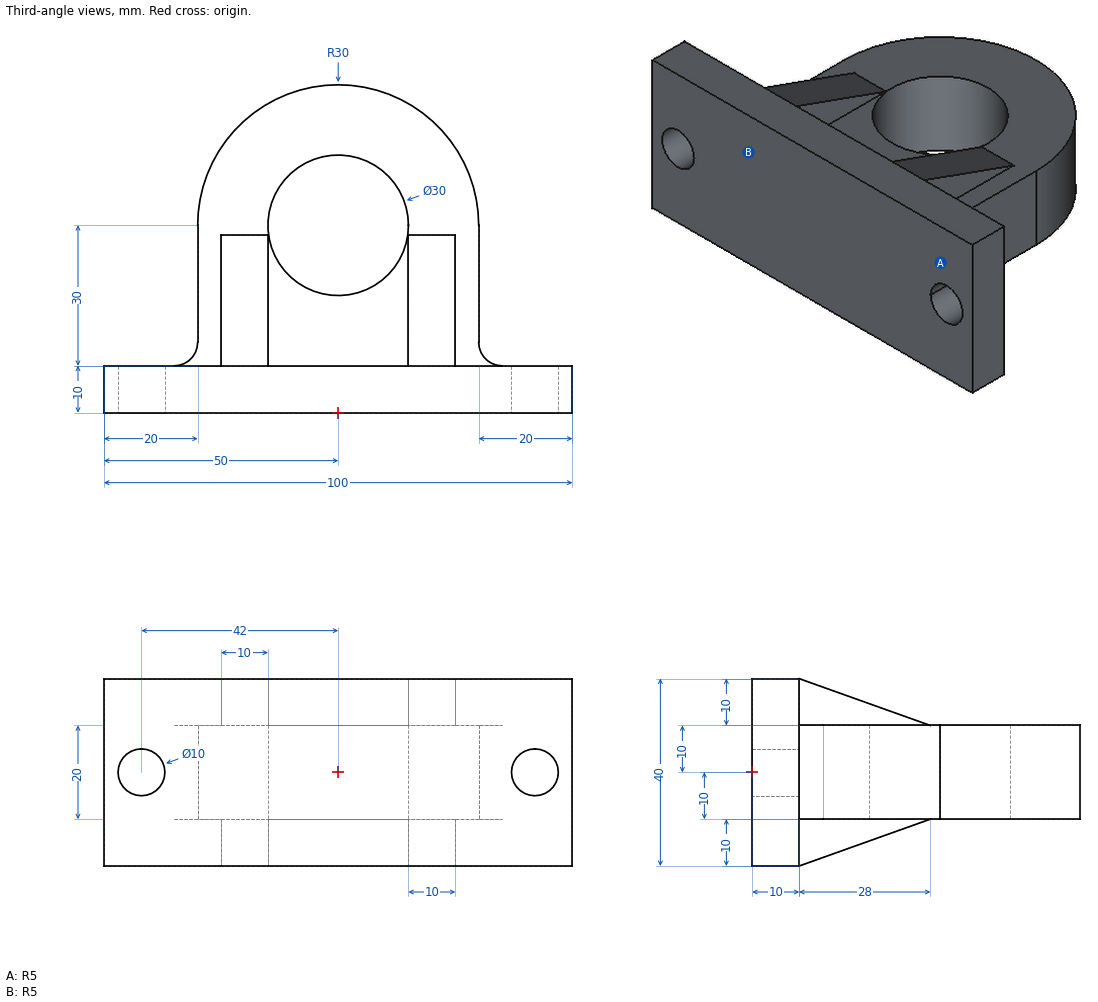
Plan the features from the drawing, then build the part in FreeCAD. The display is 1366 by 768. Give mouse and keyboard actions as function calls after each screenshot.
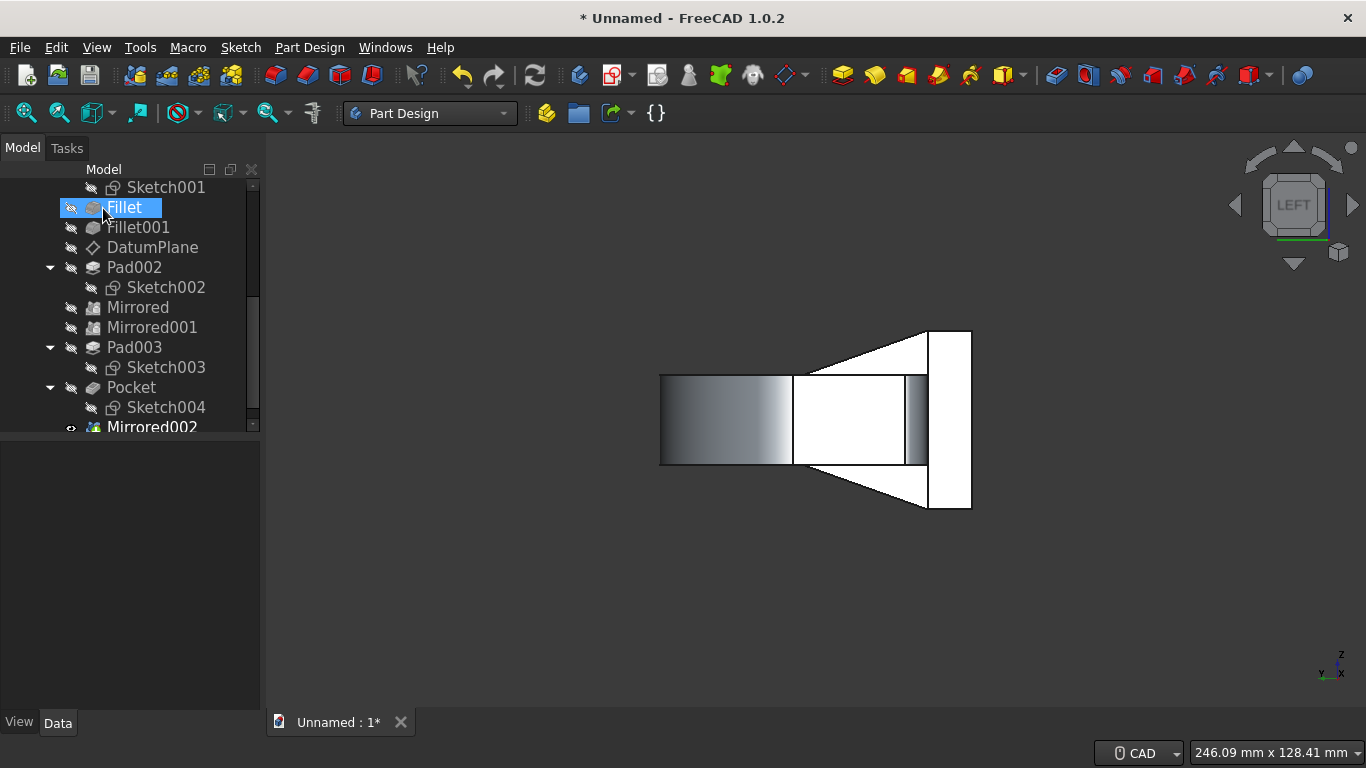
key(0)